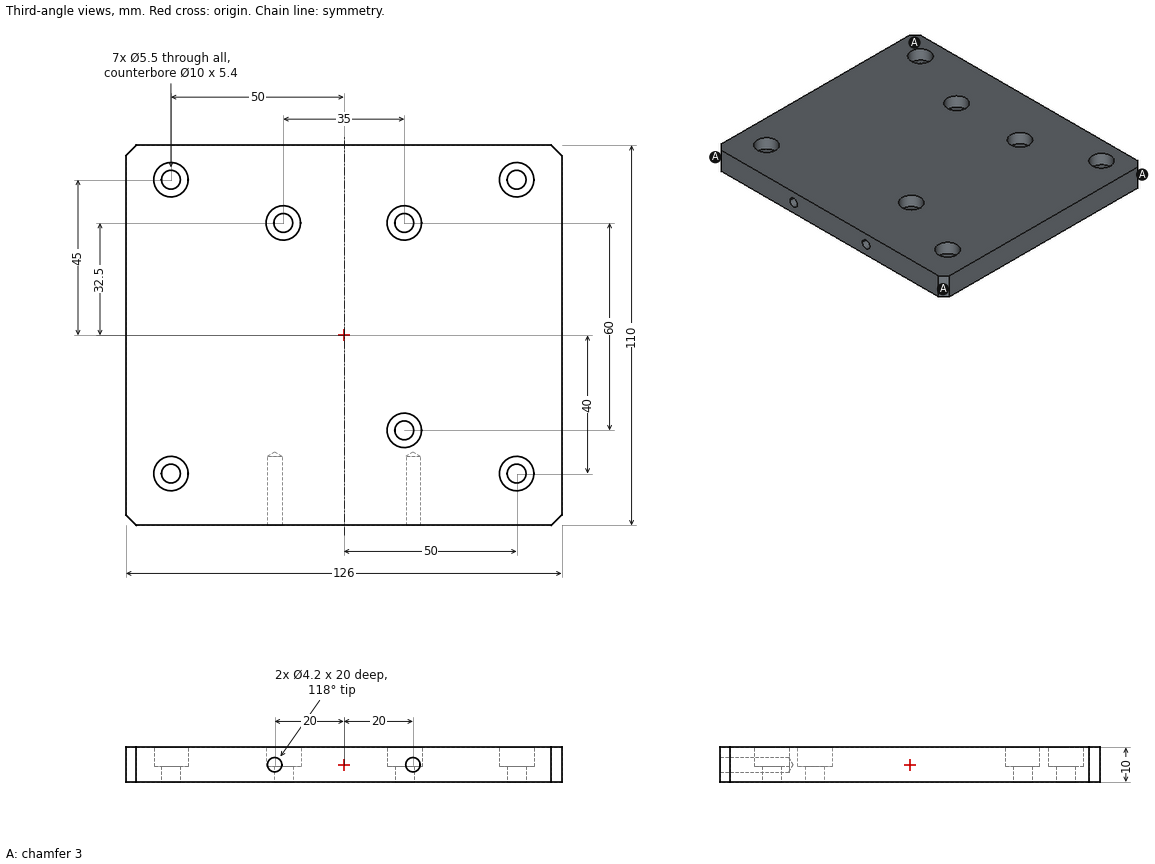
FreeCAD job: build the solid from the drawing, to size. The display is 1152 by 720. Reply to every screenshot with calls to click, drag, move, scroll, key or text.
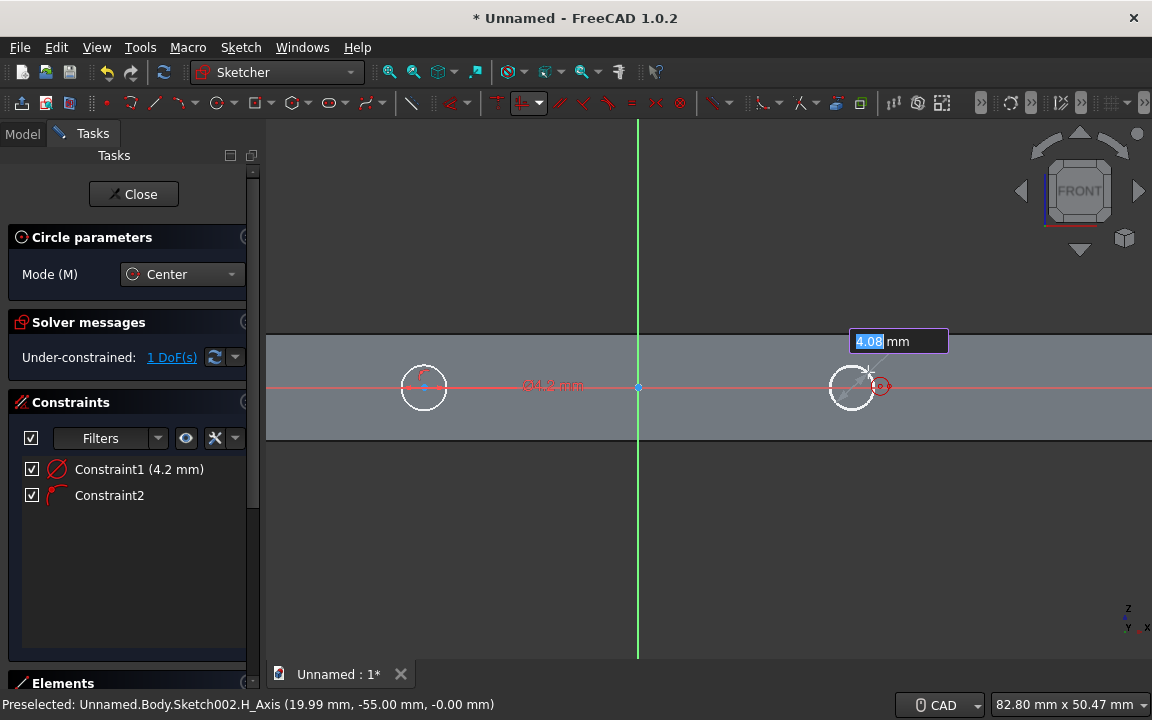
text(4.2)
key(Return)
key(Escape)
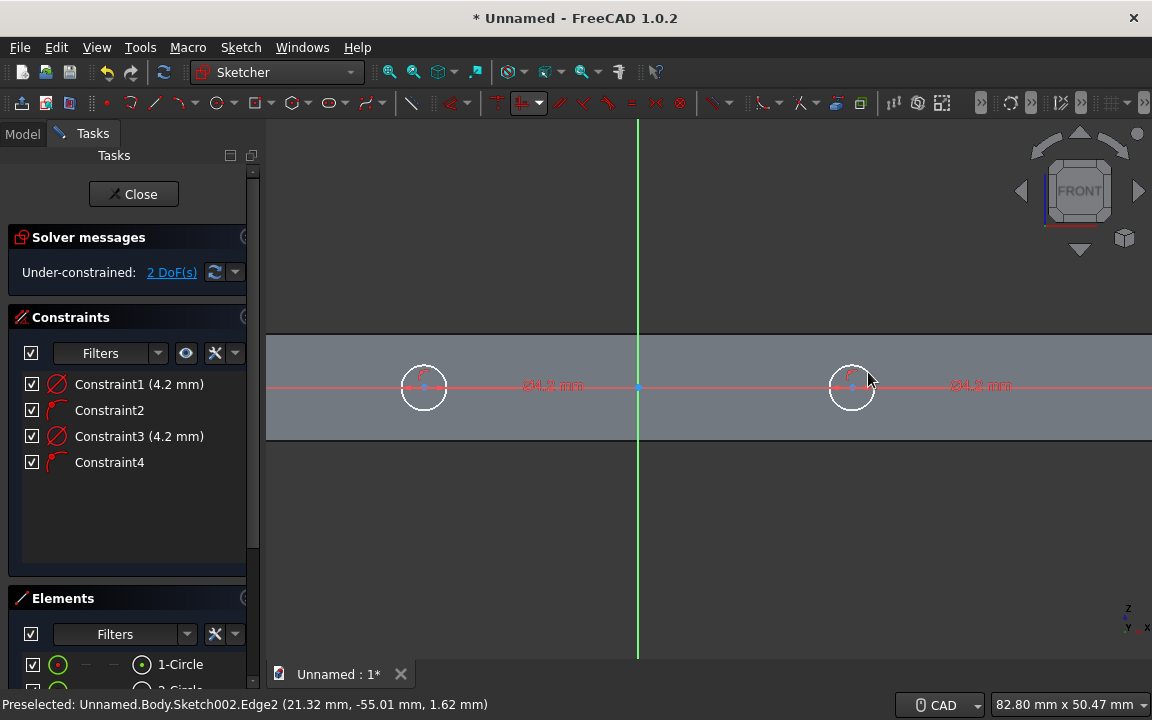
click(450, 104)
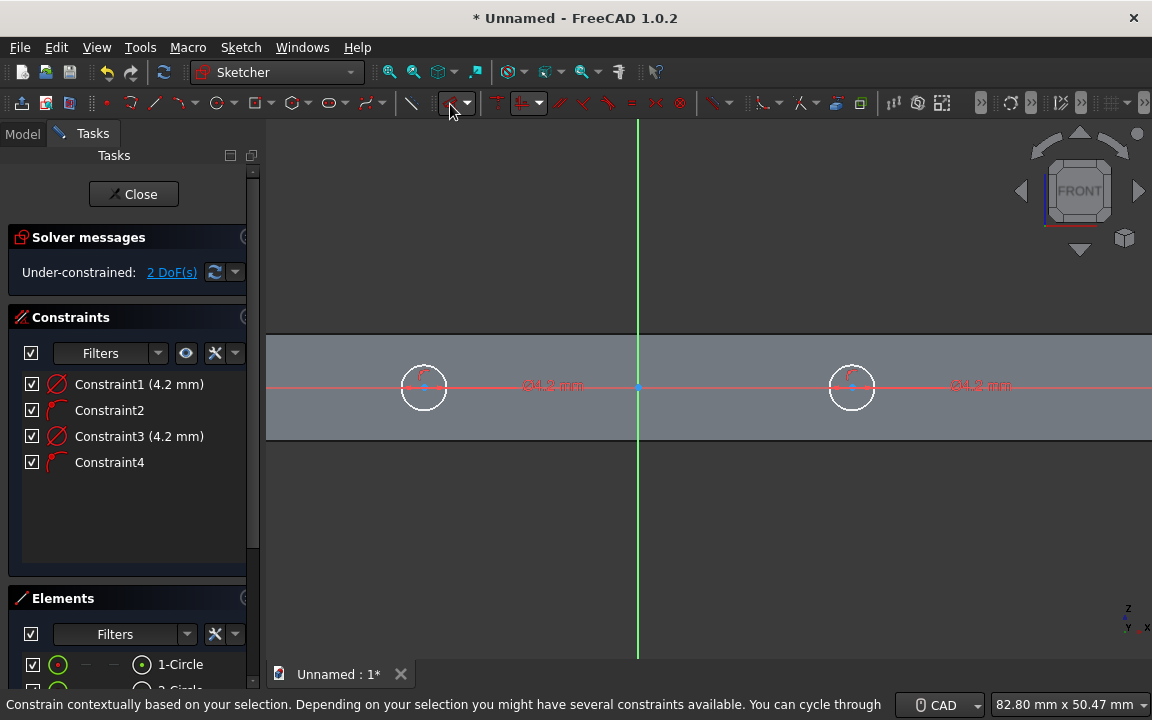
click(424, 388)
click(531, 422)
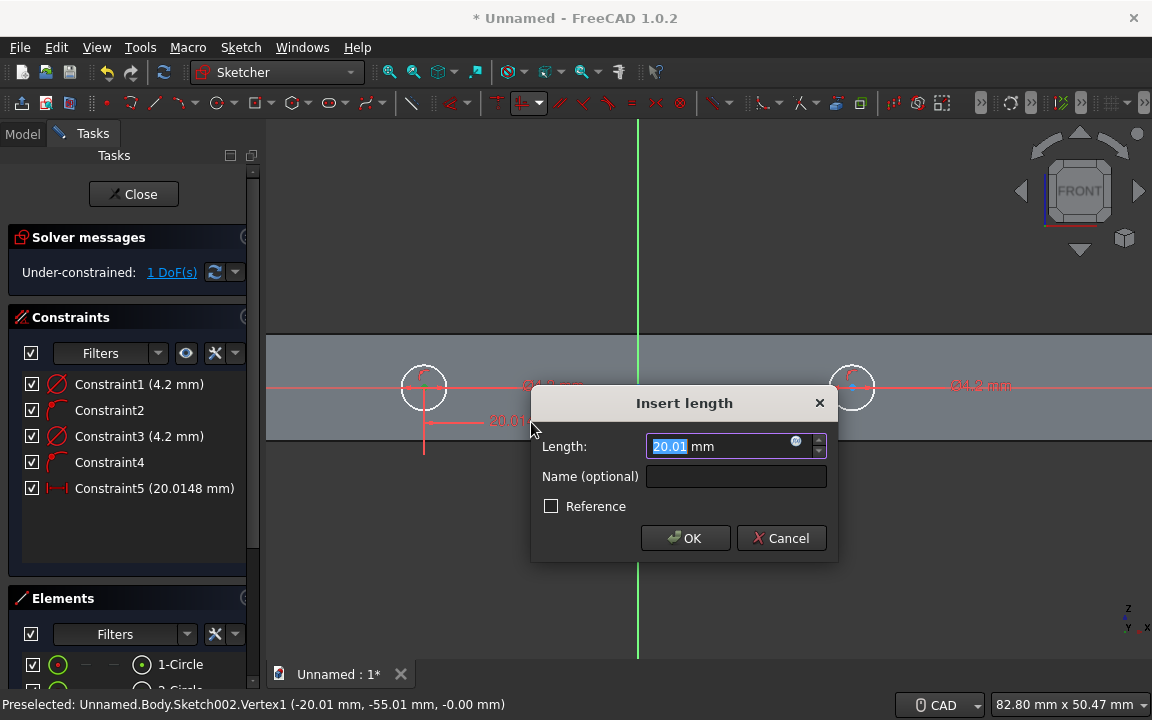
text(20)
key(Return)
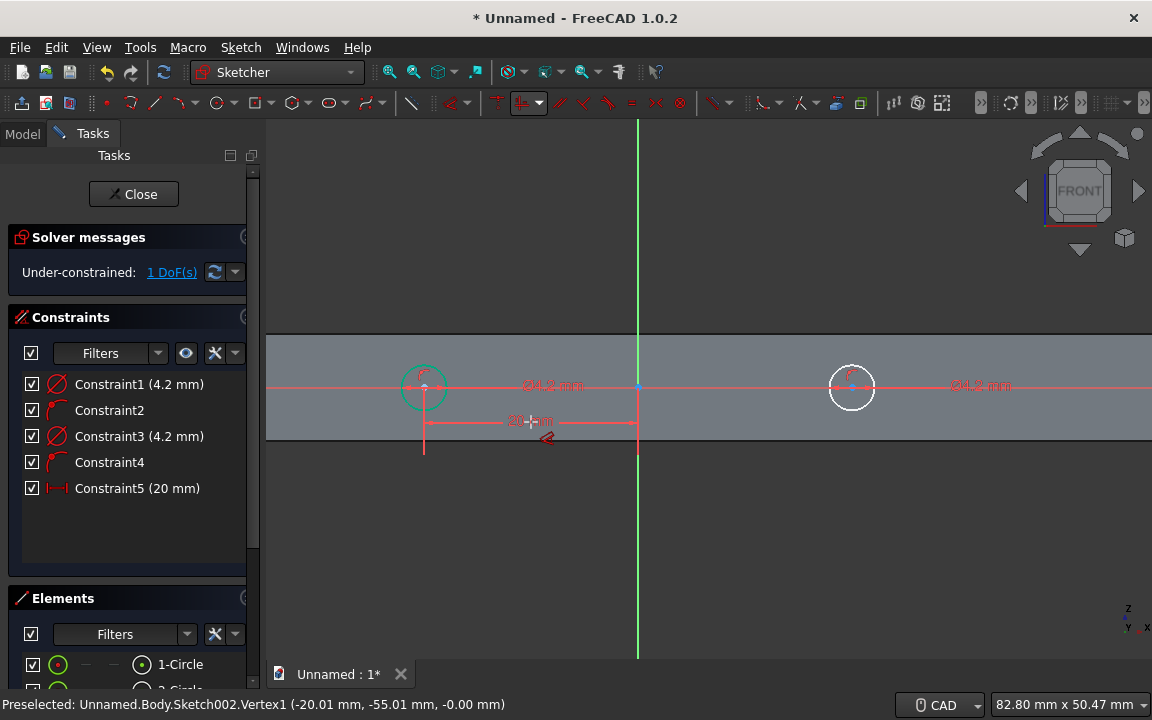
click(852, 388)
click(745, 422)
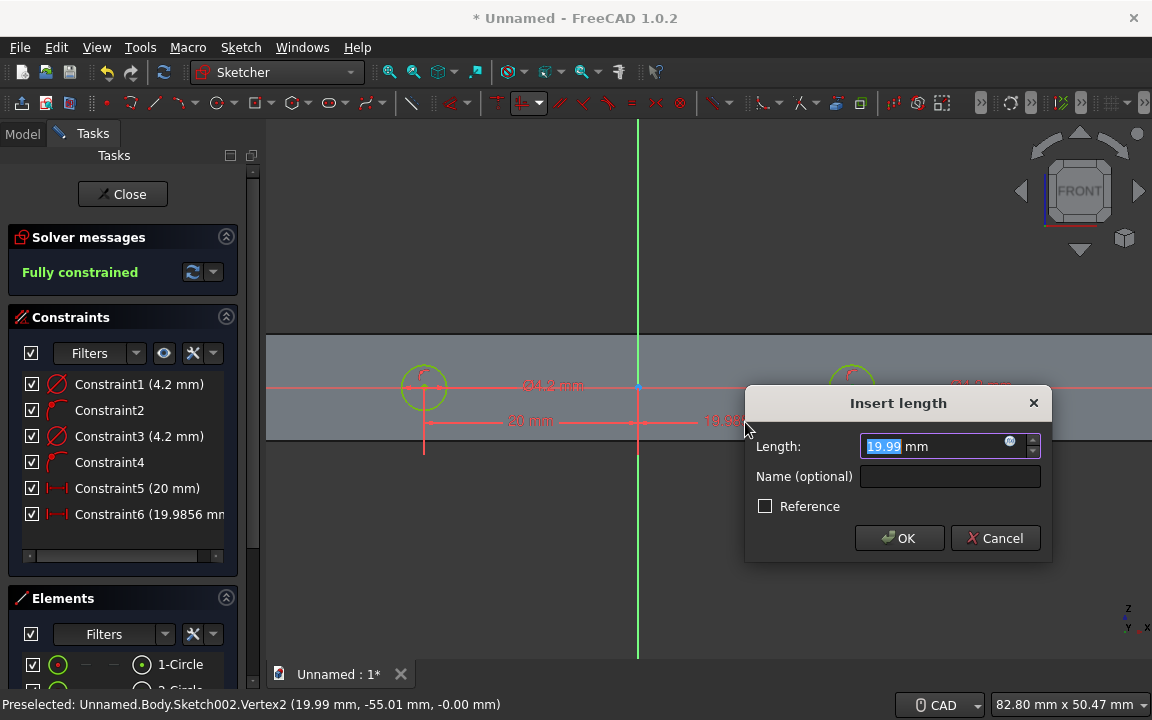
text(20)
key(Return)
key(Escape)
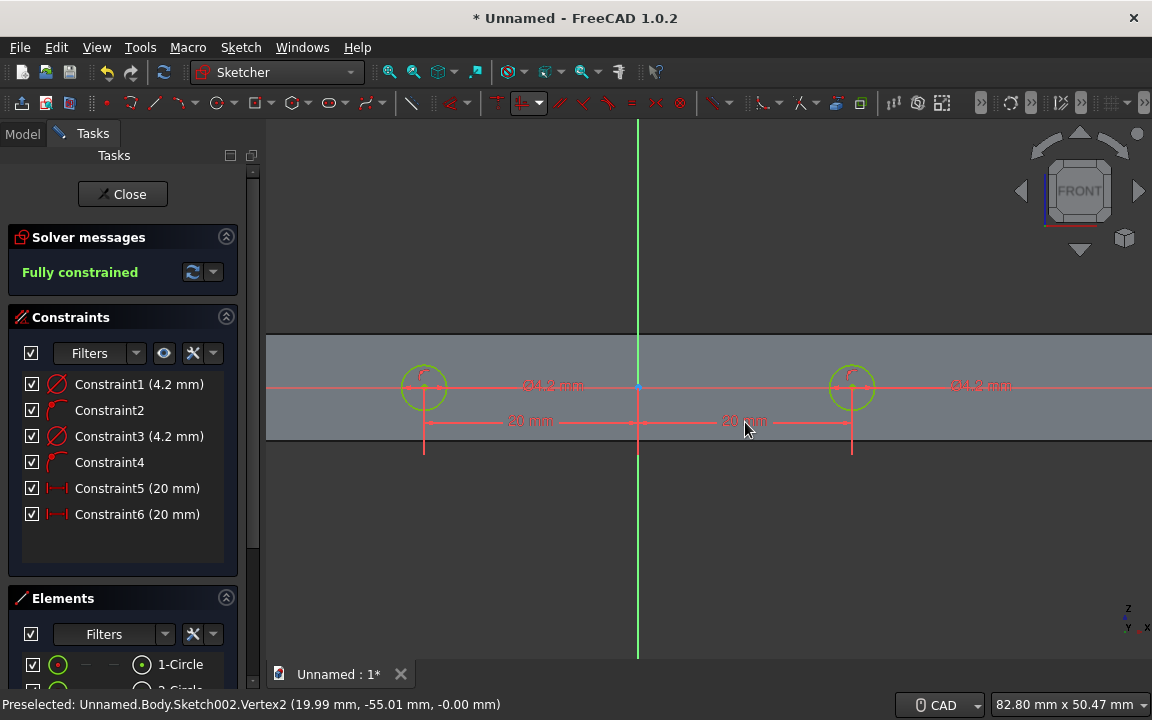
click(123, 194)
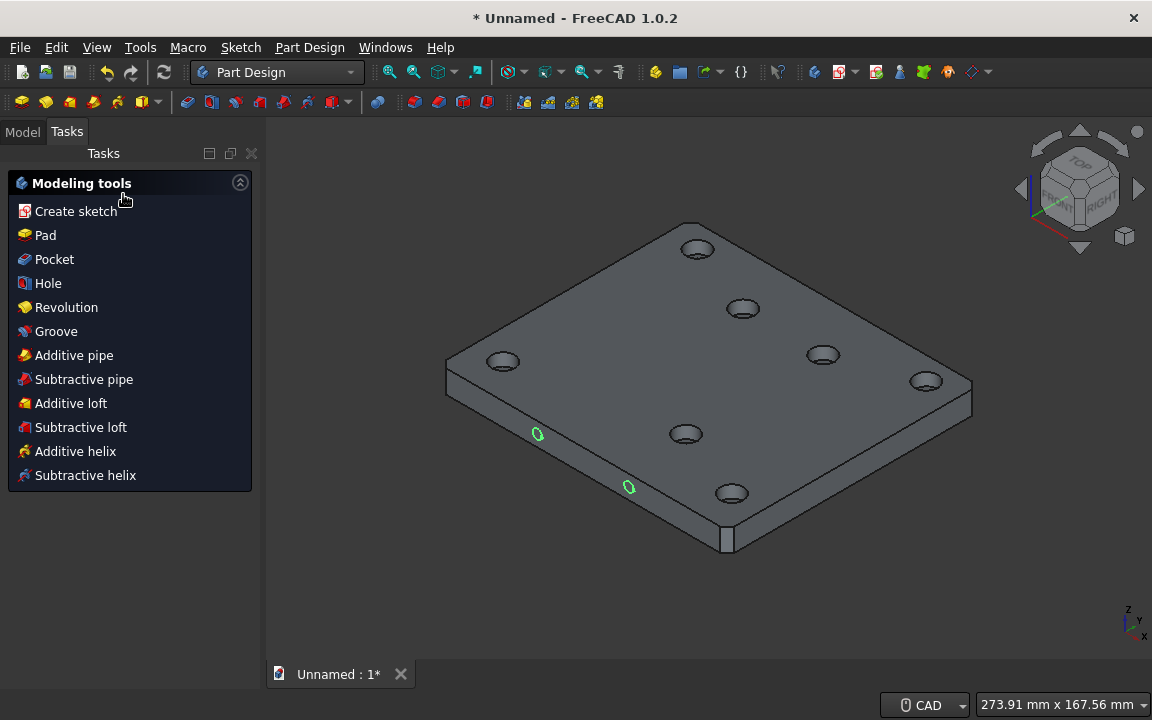
click(212, 102)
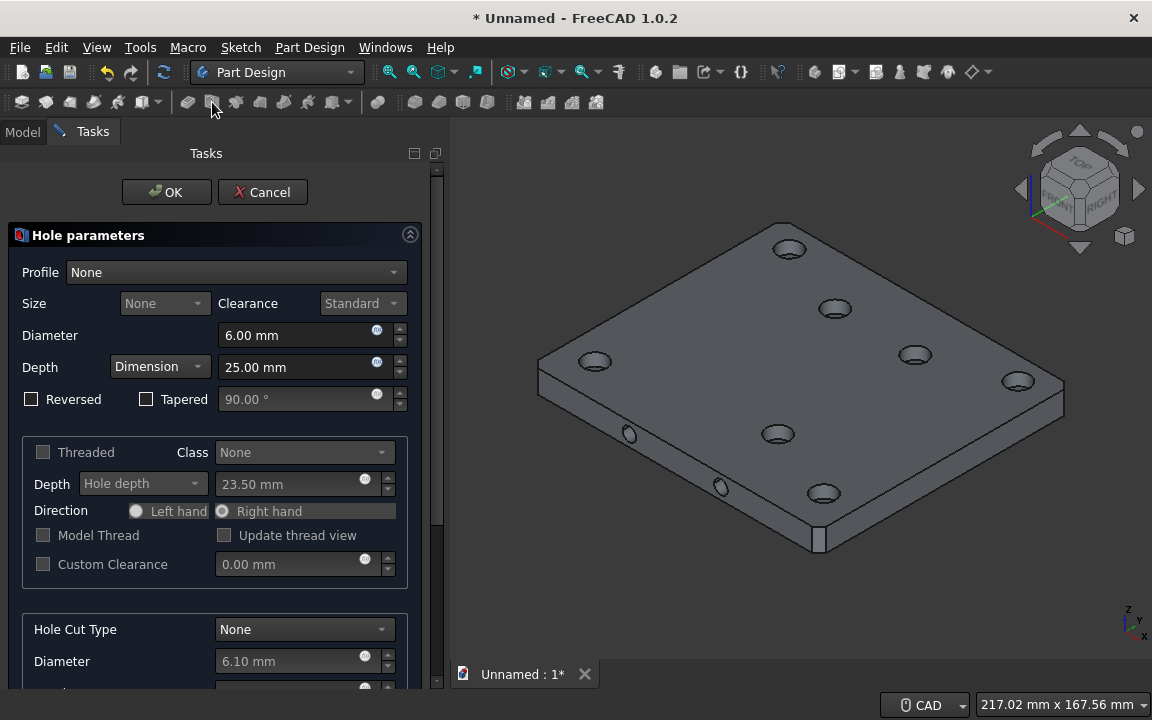
triple_click(305, 335)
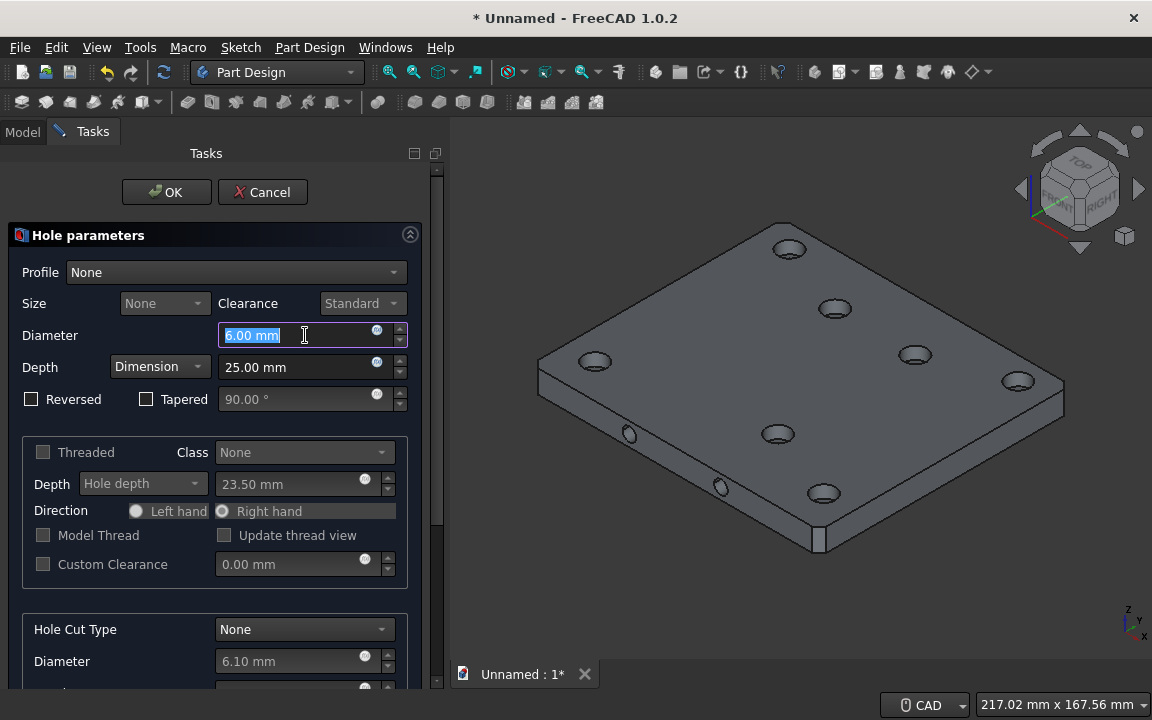
text(4.2)
key(Tab)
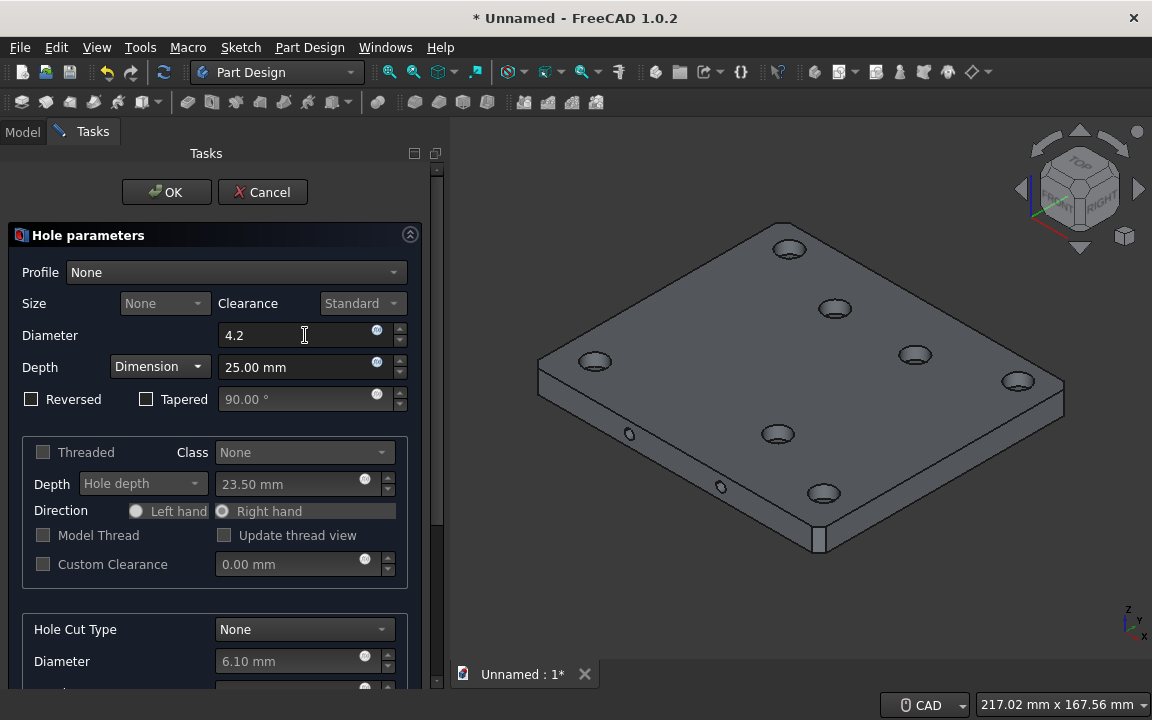
triple_click(305, 367)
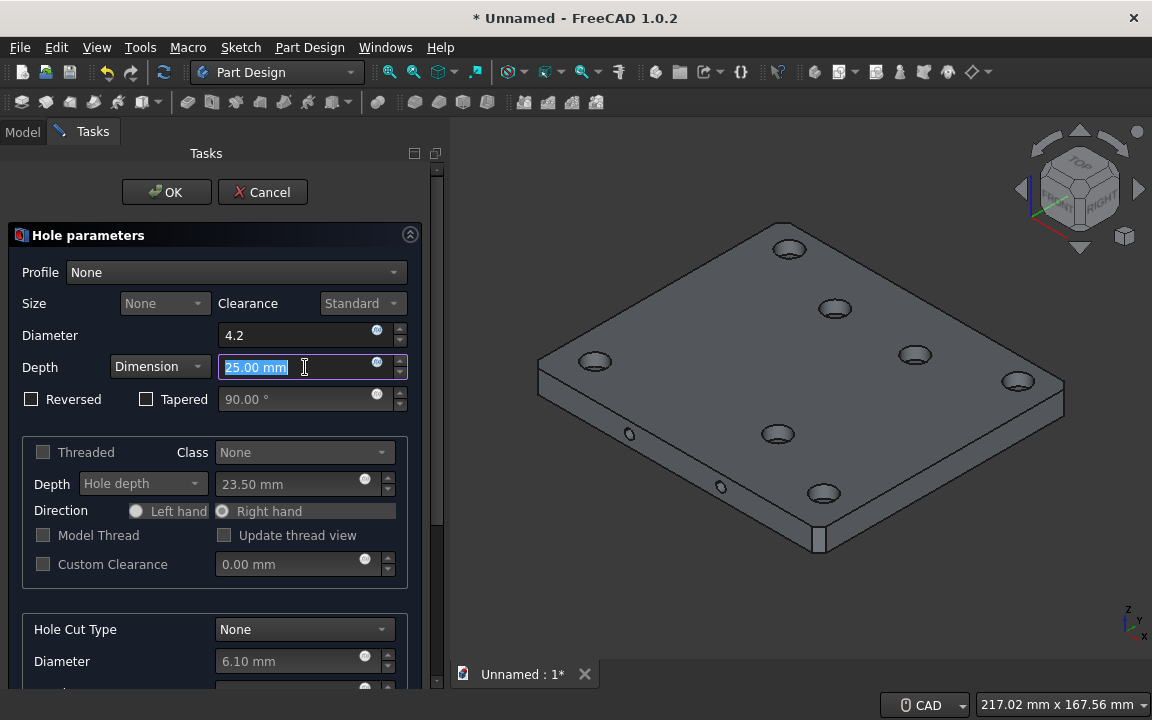
text(20)
key(Tab)